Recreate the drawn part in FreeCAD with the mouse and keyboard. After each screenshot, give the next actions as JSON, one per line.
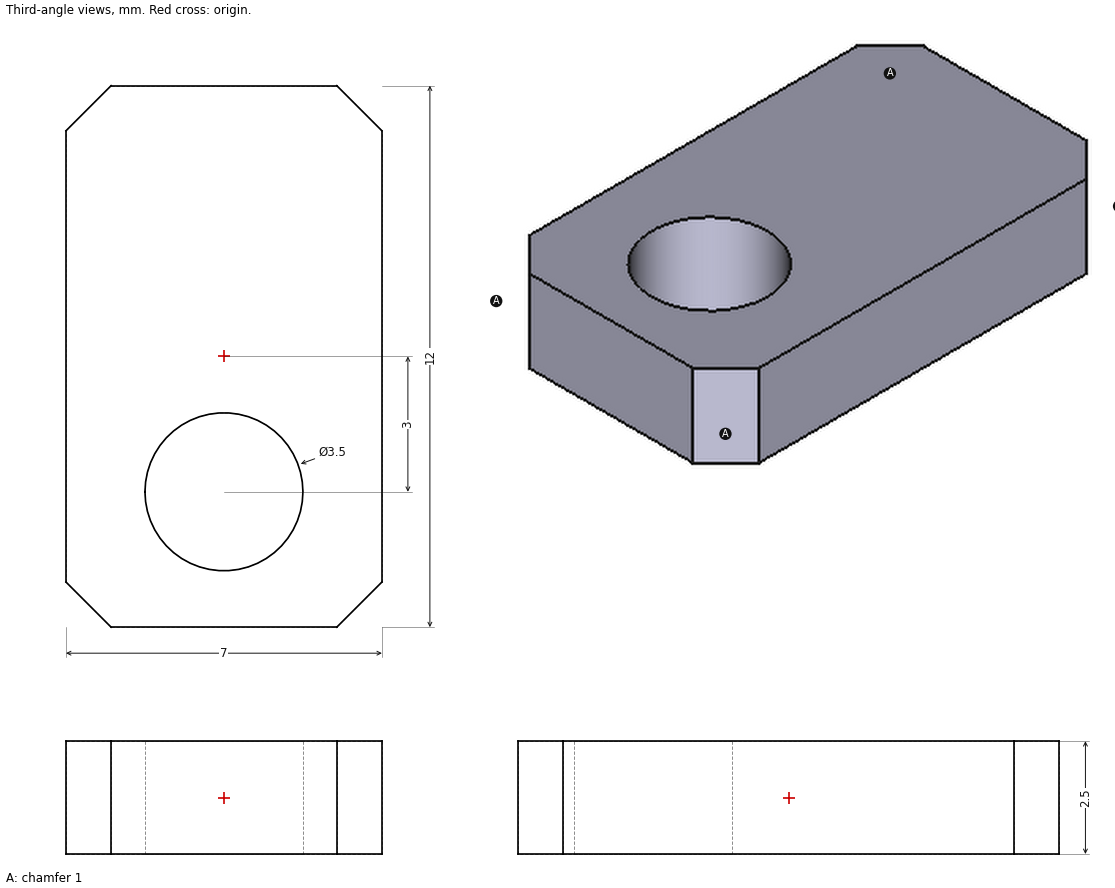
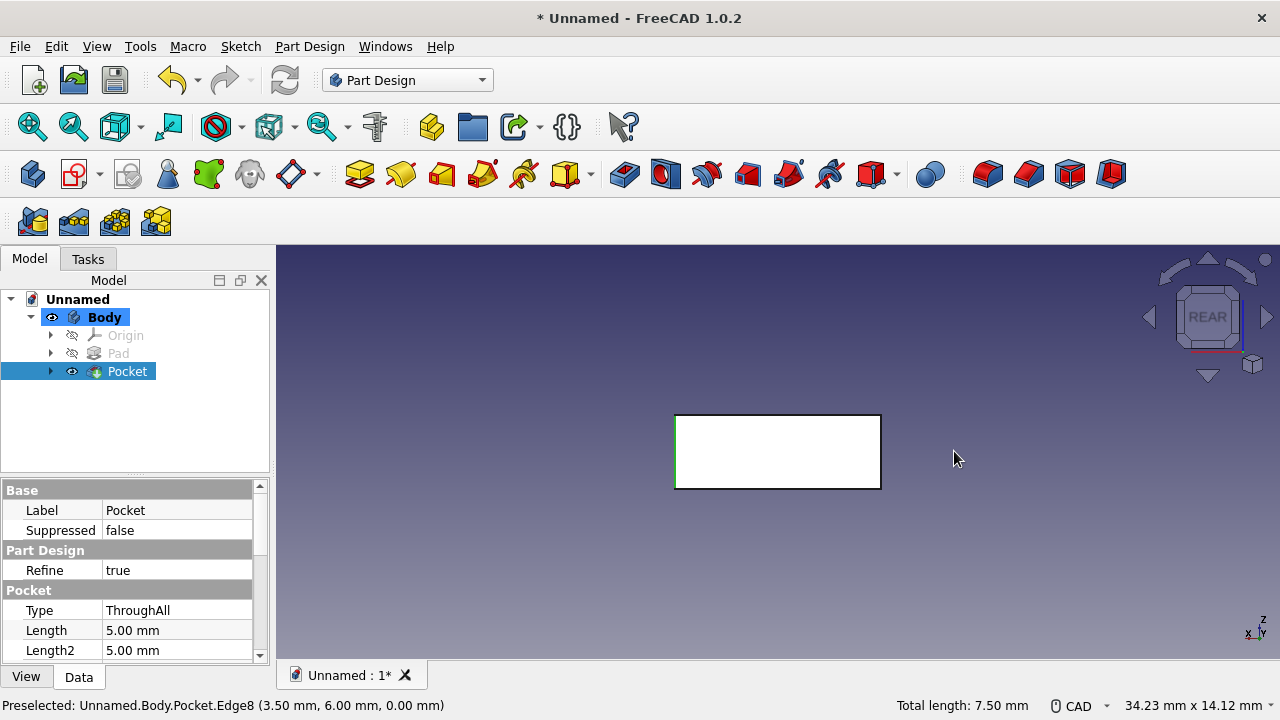
{"action": "left_click", "coordinate": [33, 128]}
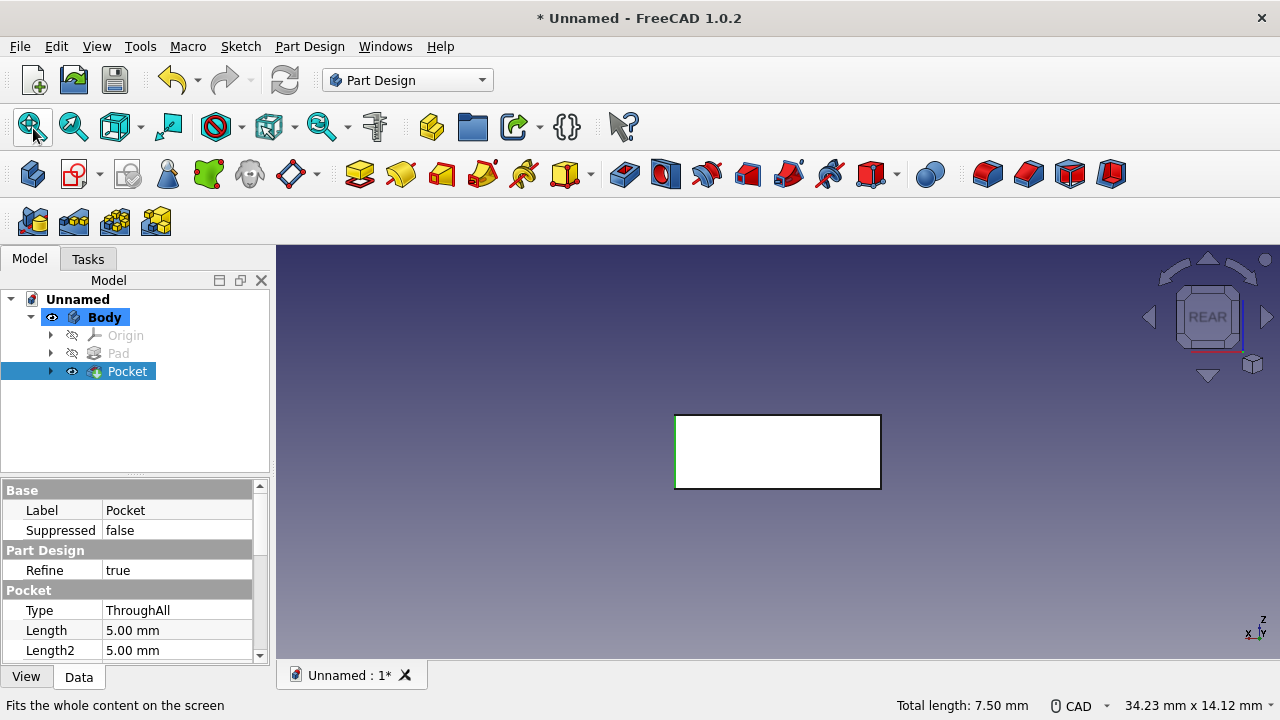
{"action": "left_click", "coordinate": [881, 451], "text": "ctrl"}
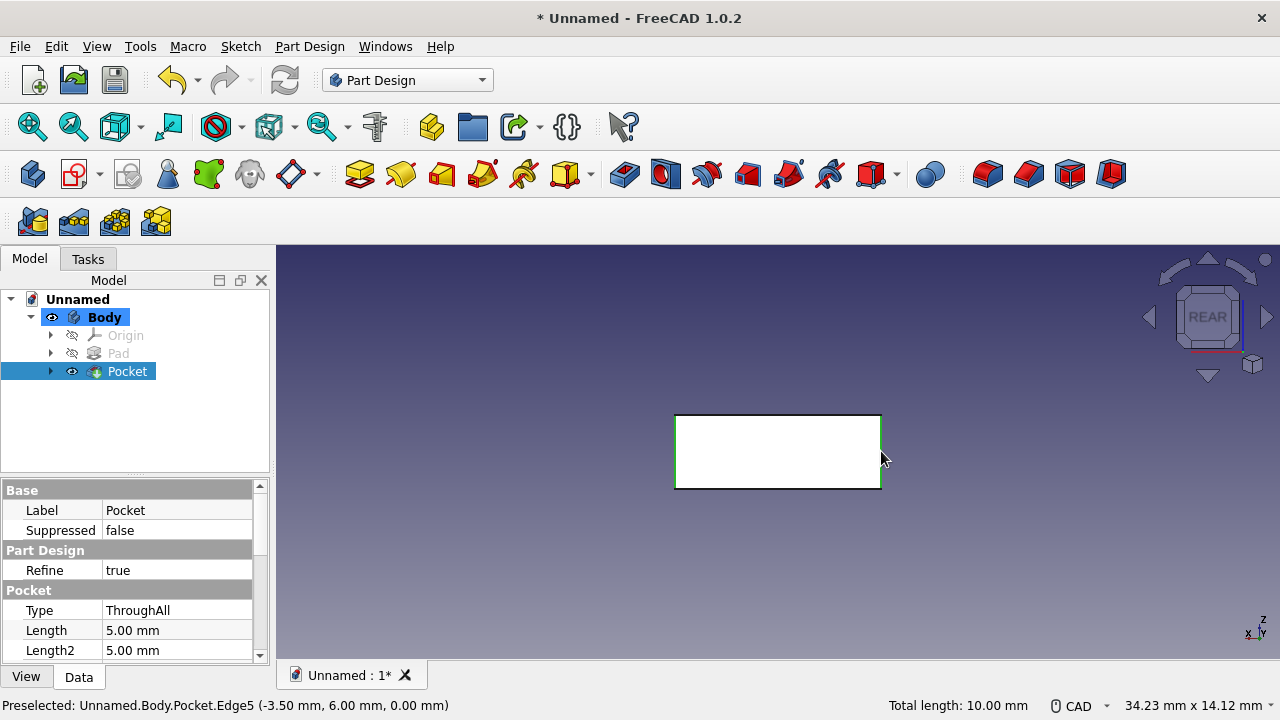
{"action": "left_click", "coordinate": [1029, 174]}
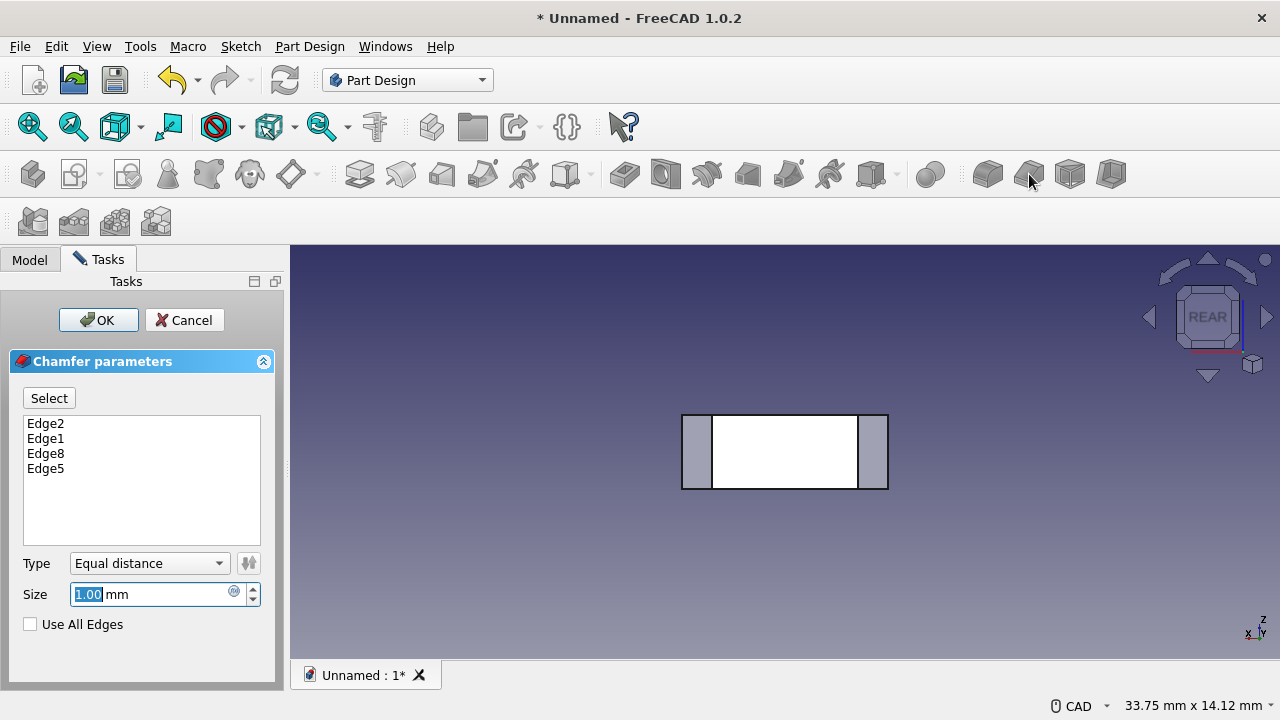
{"action": "type", "text": "1"}
{"action": "key", "text": "Tab"}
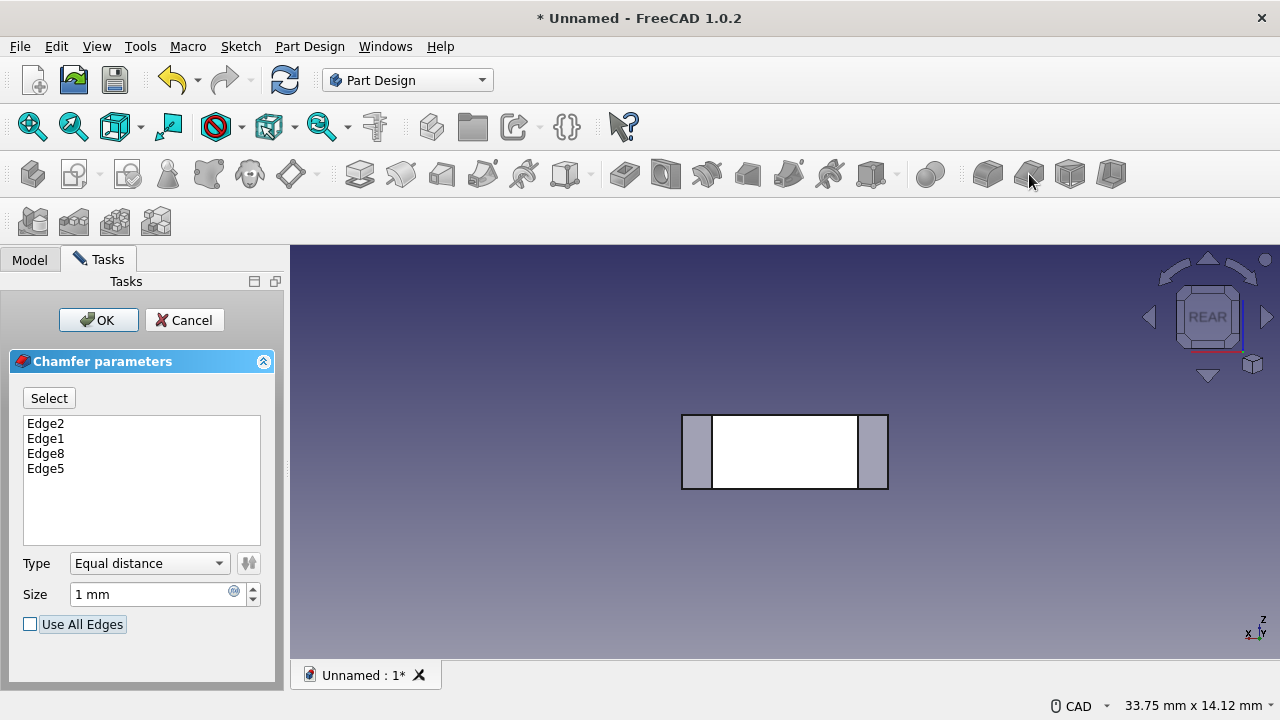
{"action": "left_click", "coordinate": [99, 320]}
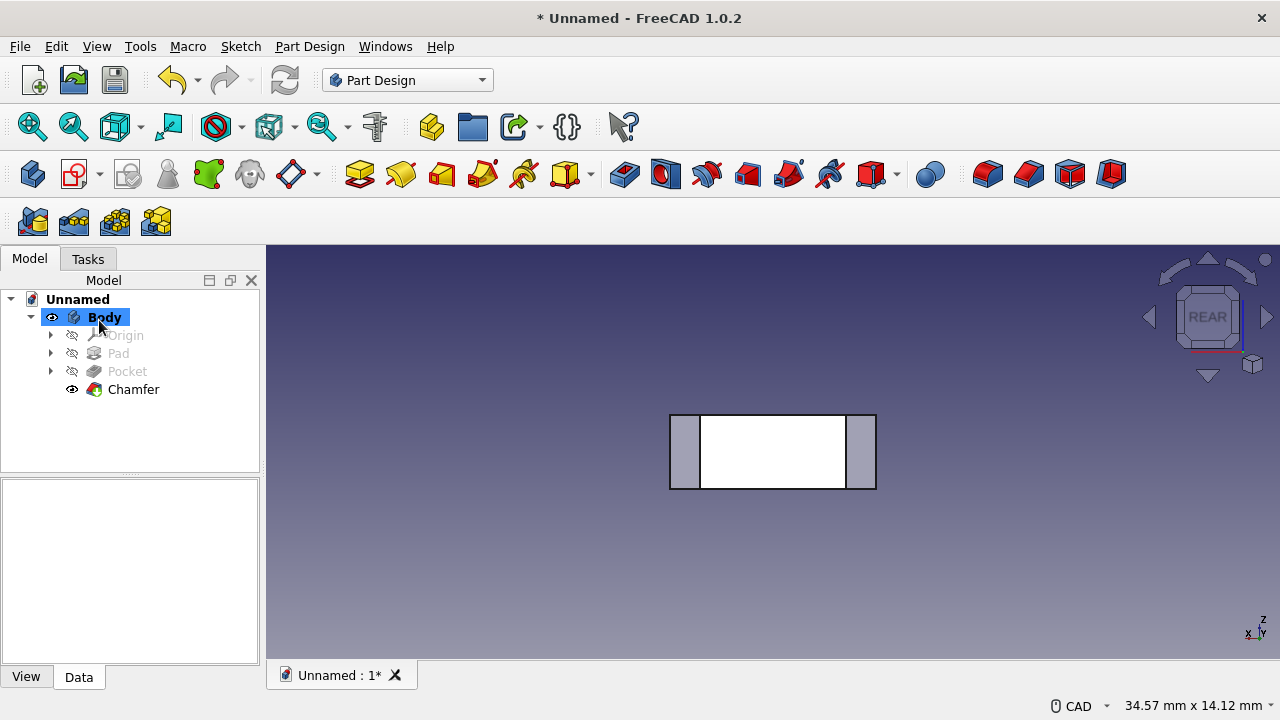
{"action": "key", "text": "0"}